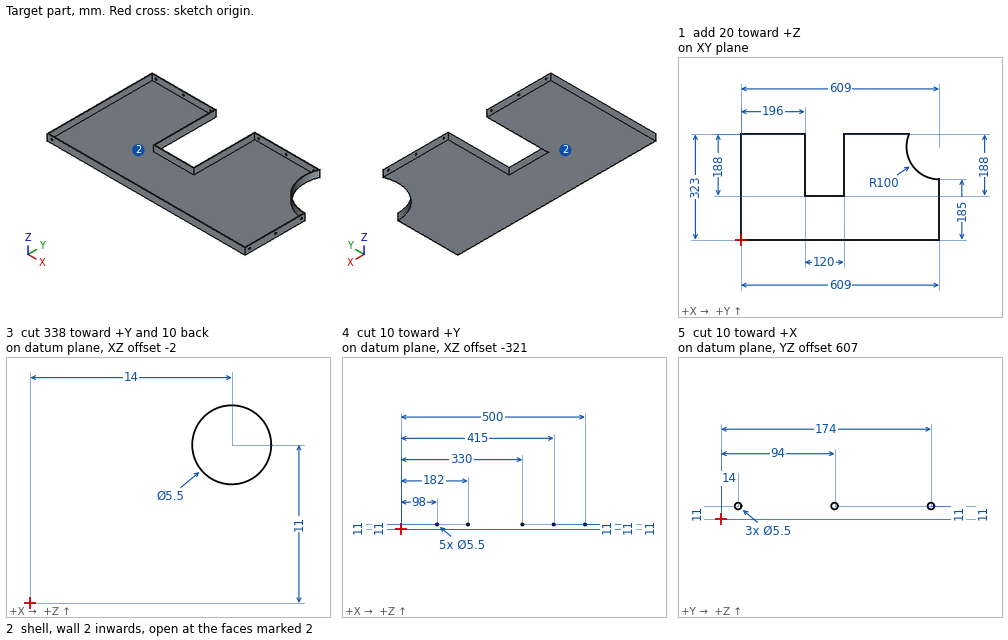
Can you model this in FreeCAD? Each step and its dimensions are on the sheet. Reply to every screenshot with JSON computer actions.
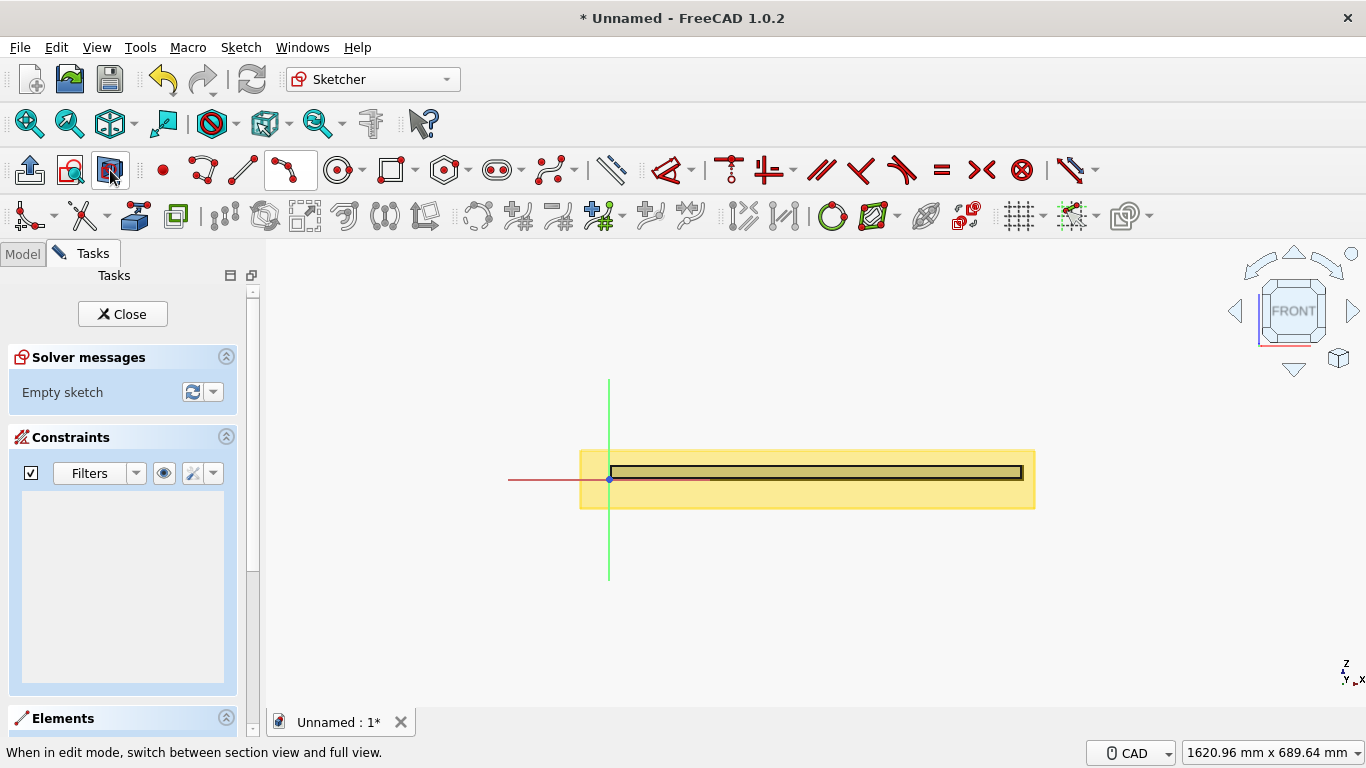
{"action": "scroll", "coordinate": [612, 472], "scroll_direction": "up", "scroll_amount": 15}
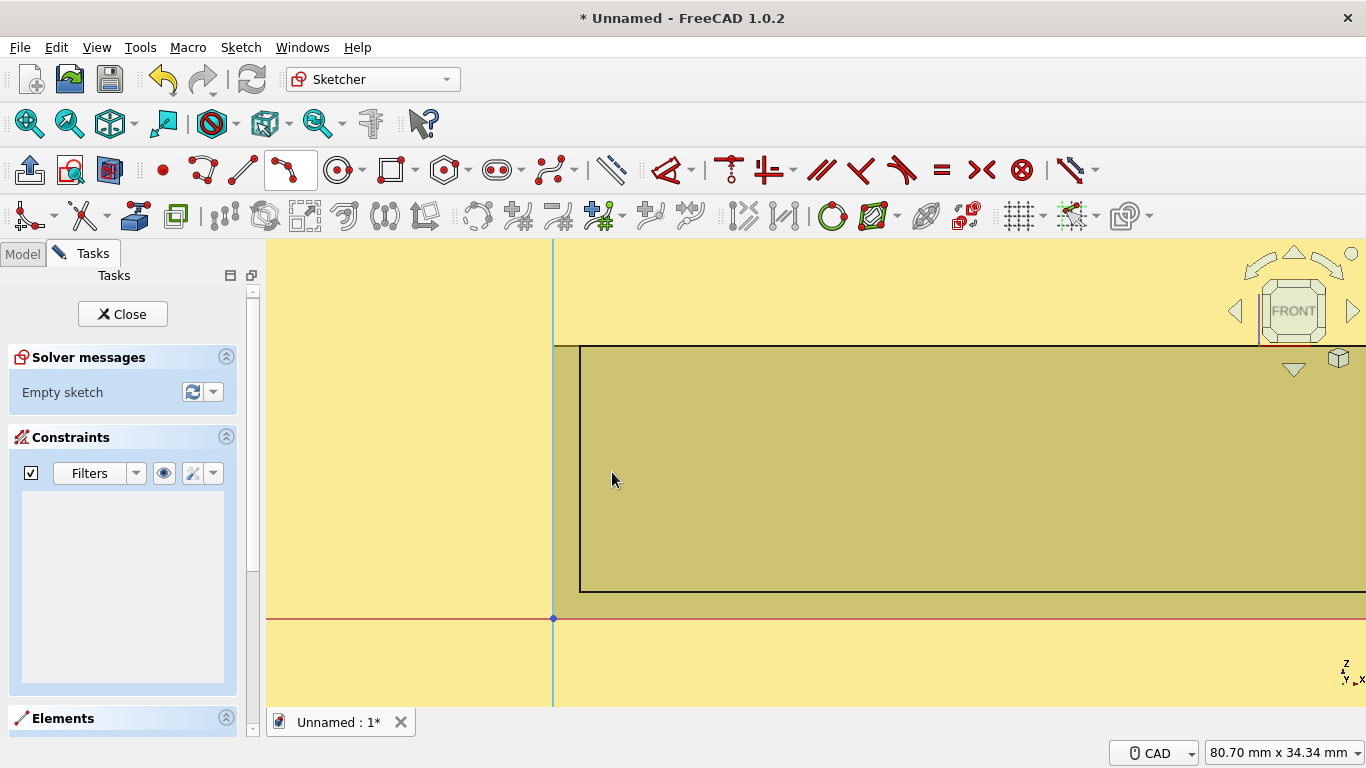
{"action": "scroll", "coordinate": [743, 468], "scroll_direction": "up", "scroll_amount": 7}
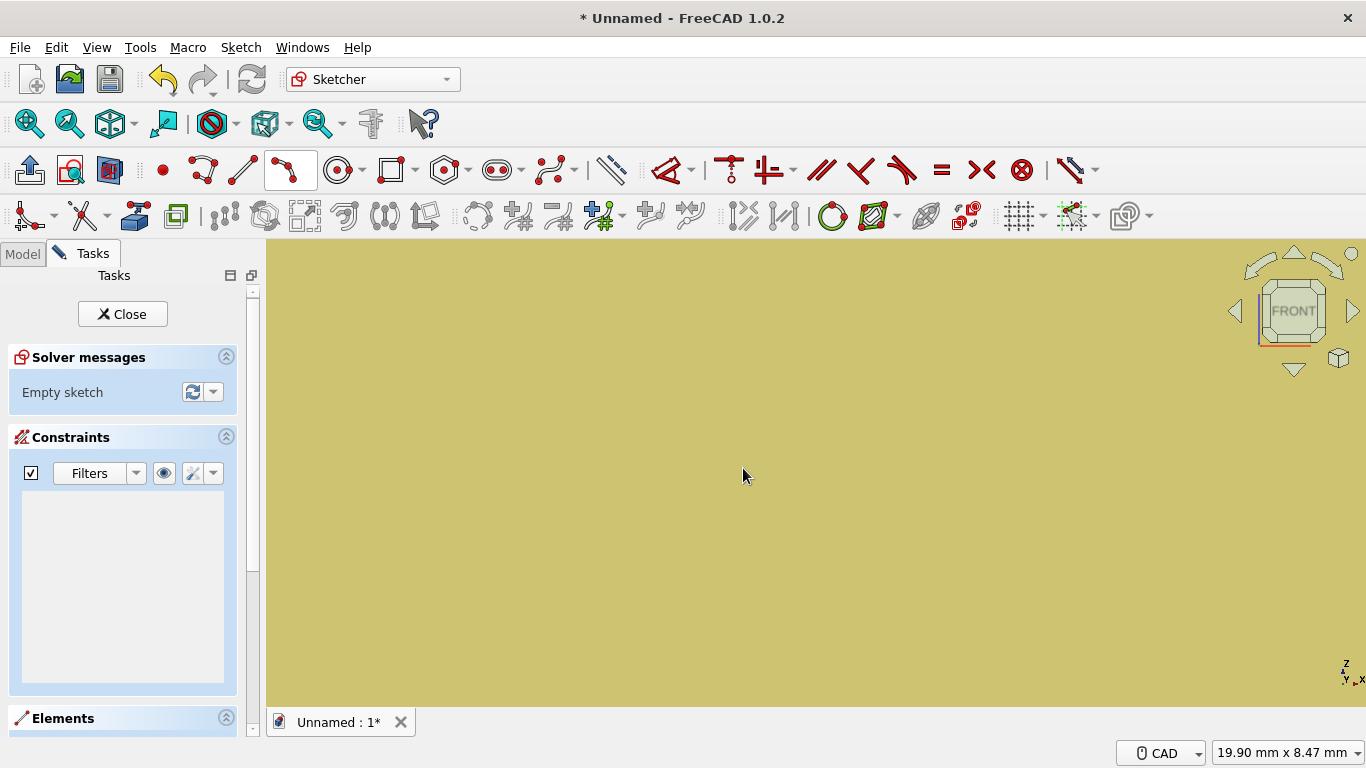
{"action": "key", "text": "g c"}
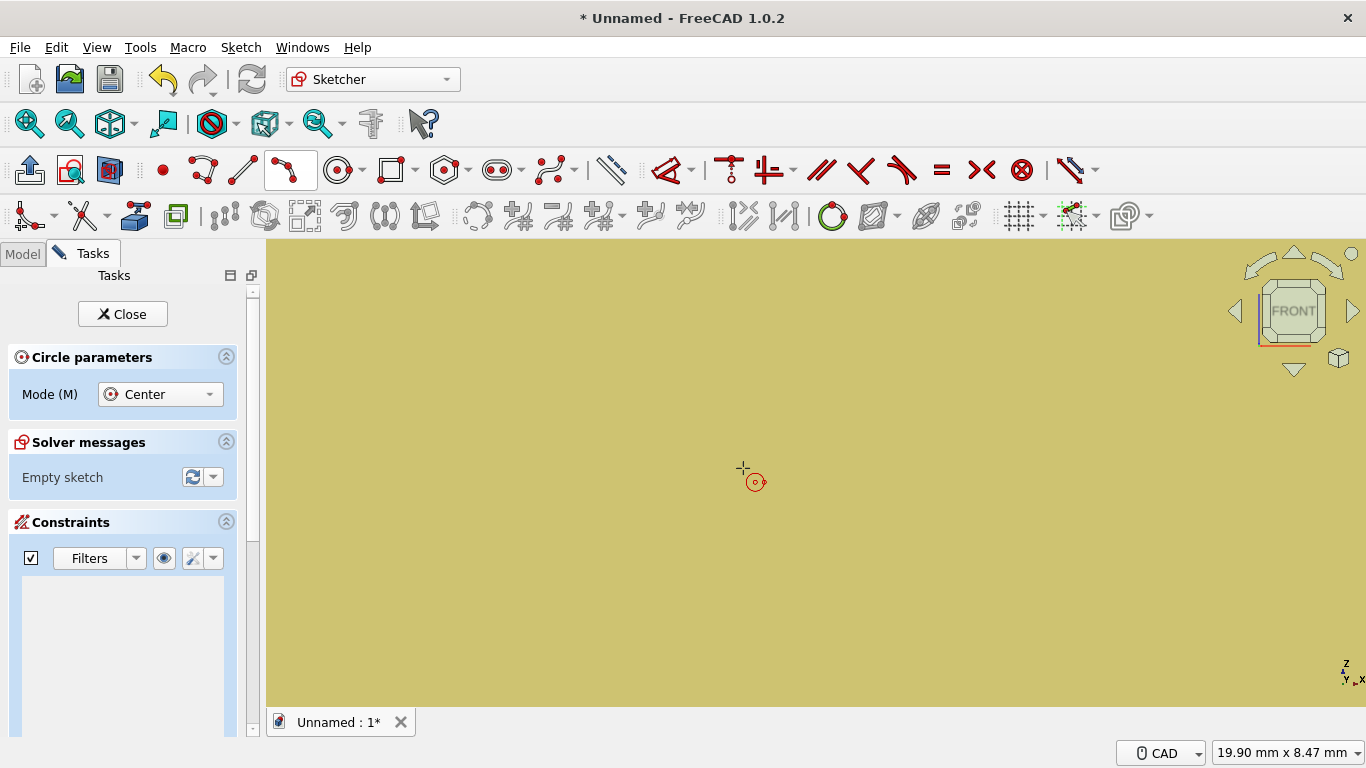
{"action": "left_click", "coordinate": [745, 470]}
{"action": "left_click", "coordinate": [853, 363]}
{"action": "key", "text": "Escape"}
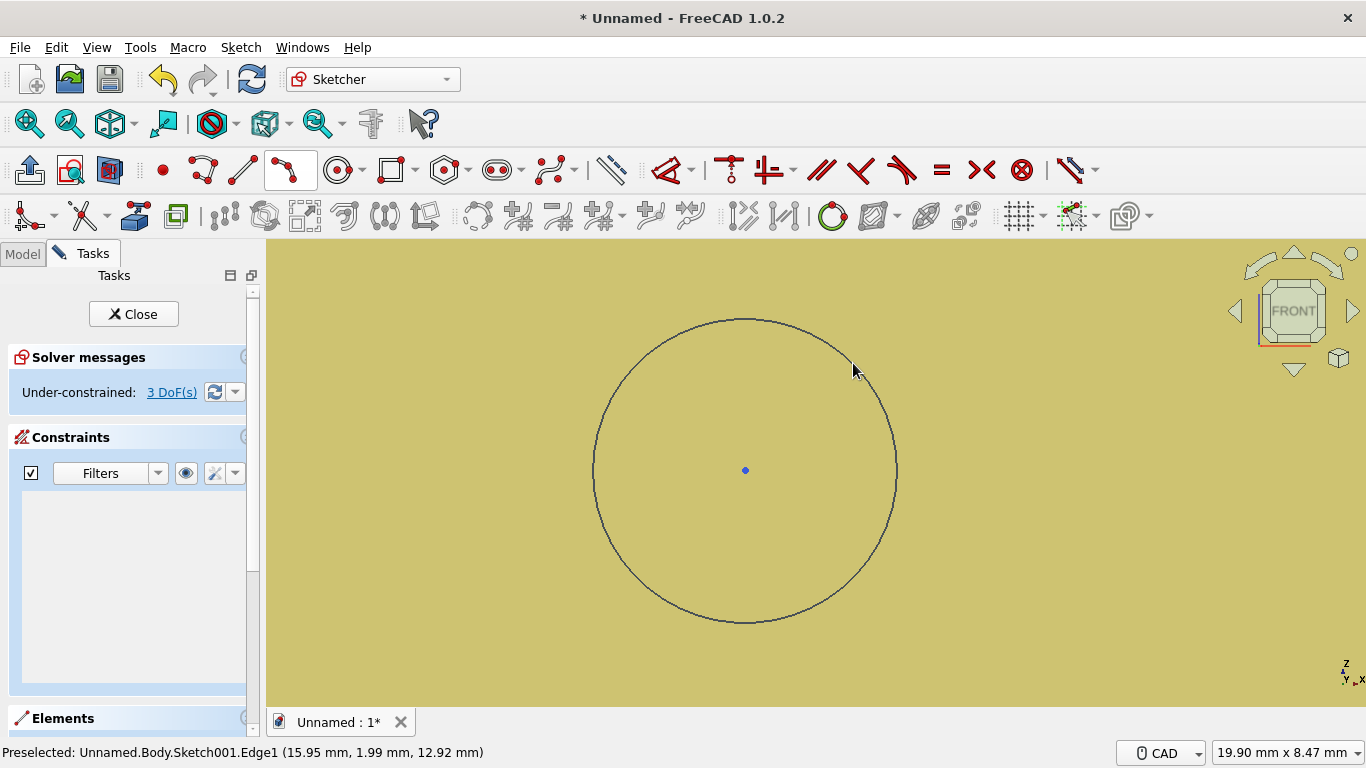
{"action": "left_click", "coordinate": [852, 363]}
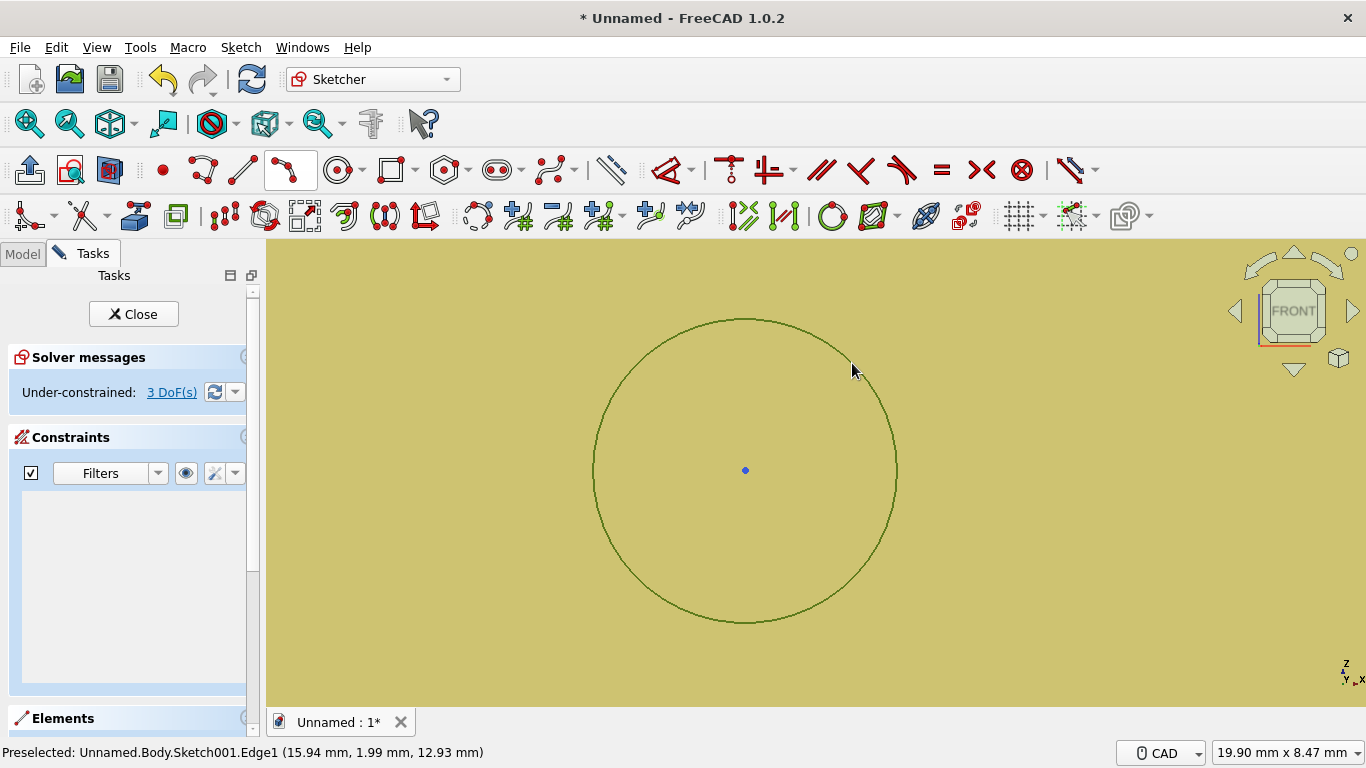
{"action": "key", "text": "k o"}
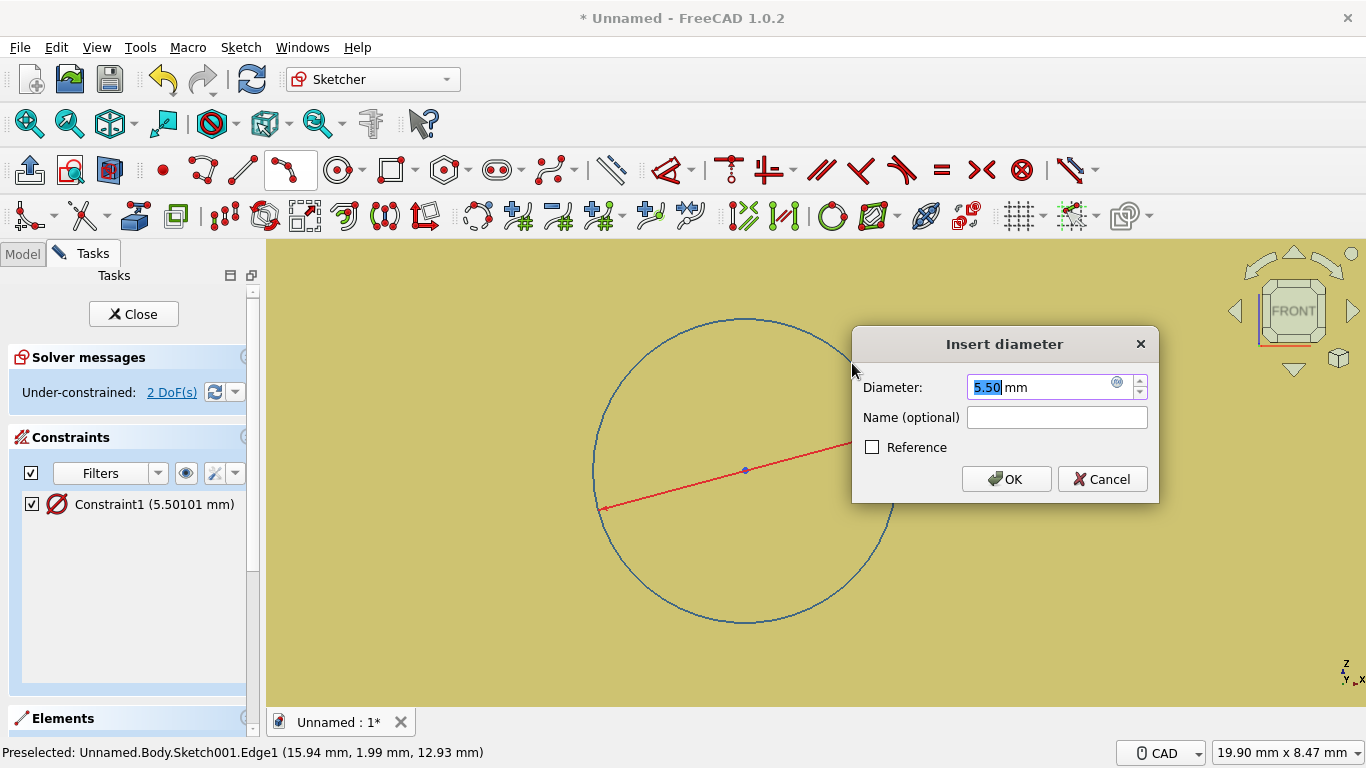
{"action": "type", "text": "5.5"}
{"action": "key", "text": "Return"}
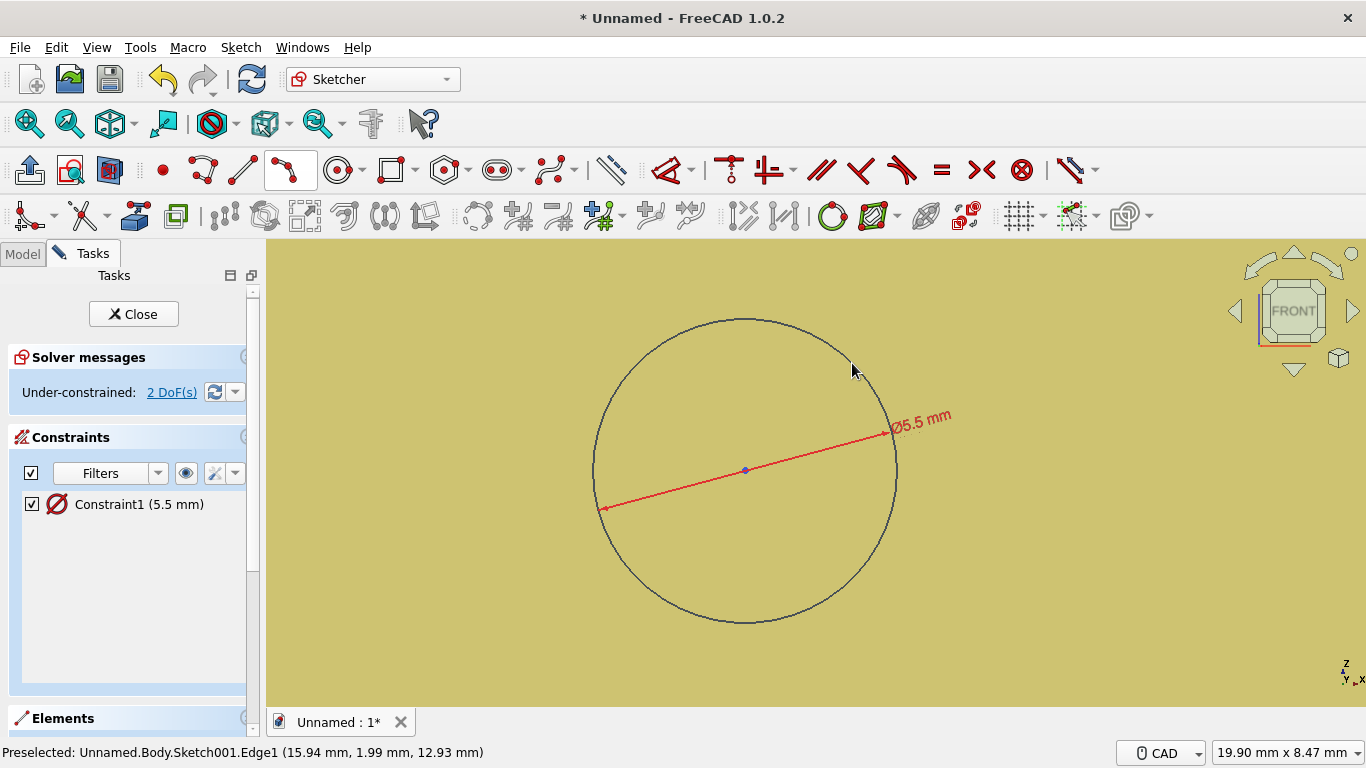
{"action": "left_click", "coordinate": [745, 471]}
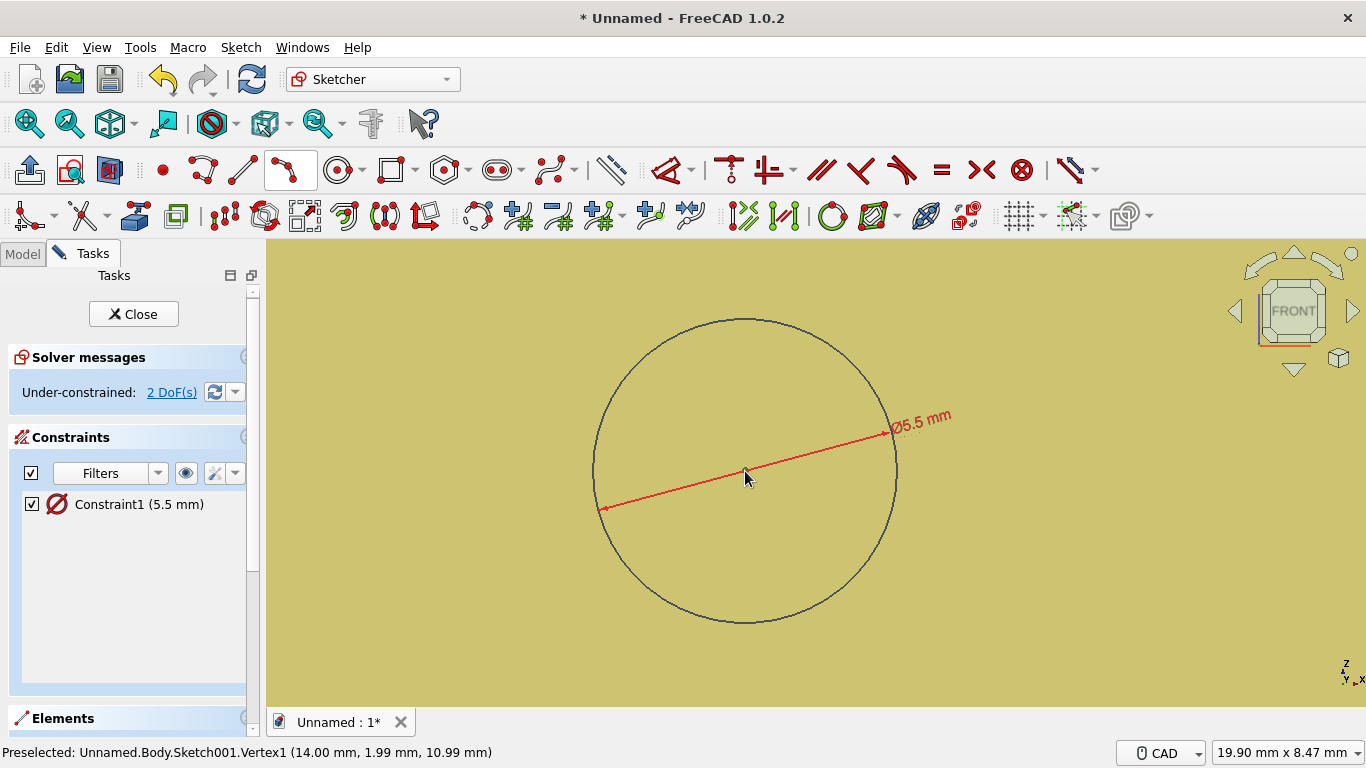
{"action": "key", "text": "l"}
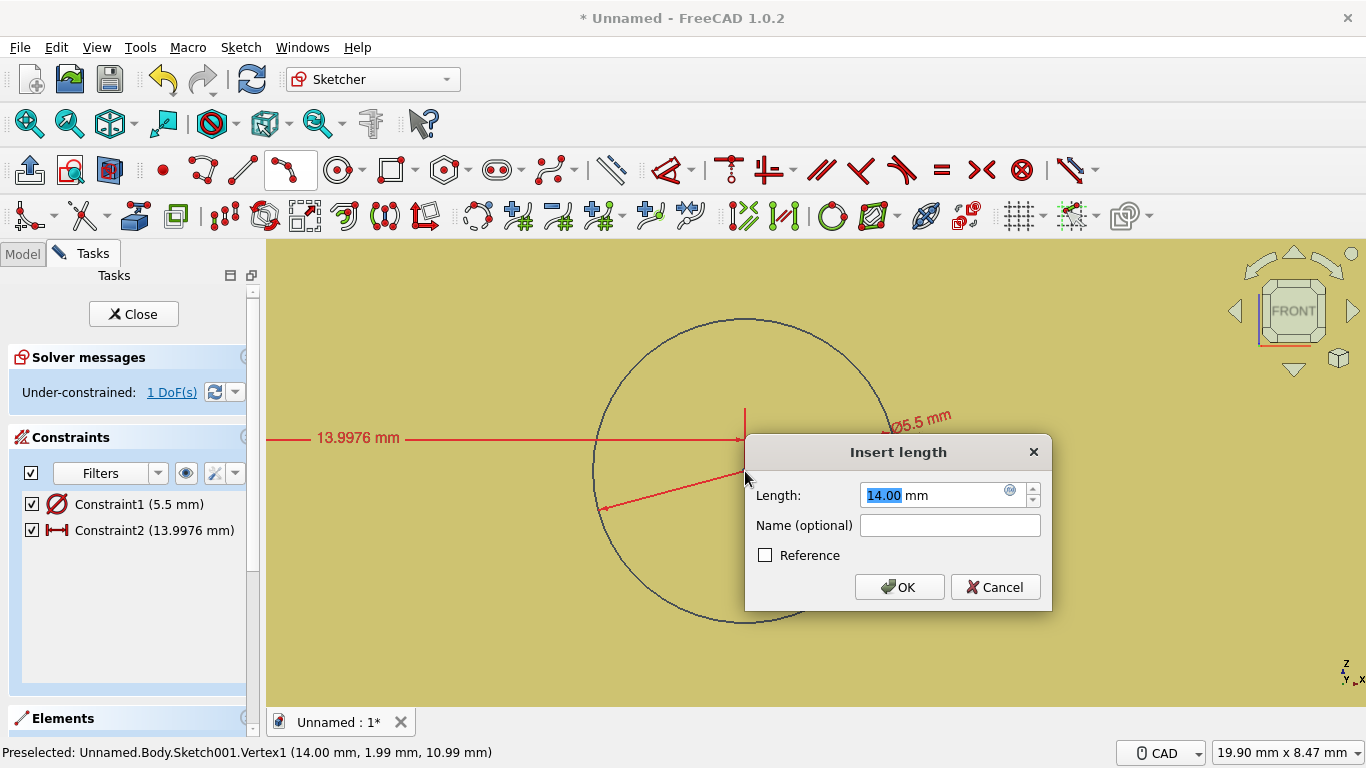
{"action": "type", "text": "14"}
{"action": "key", "text": "Return"}